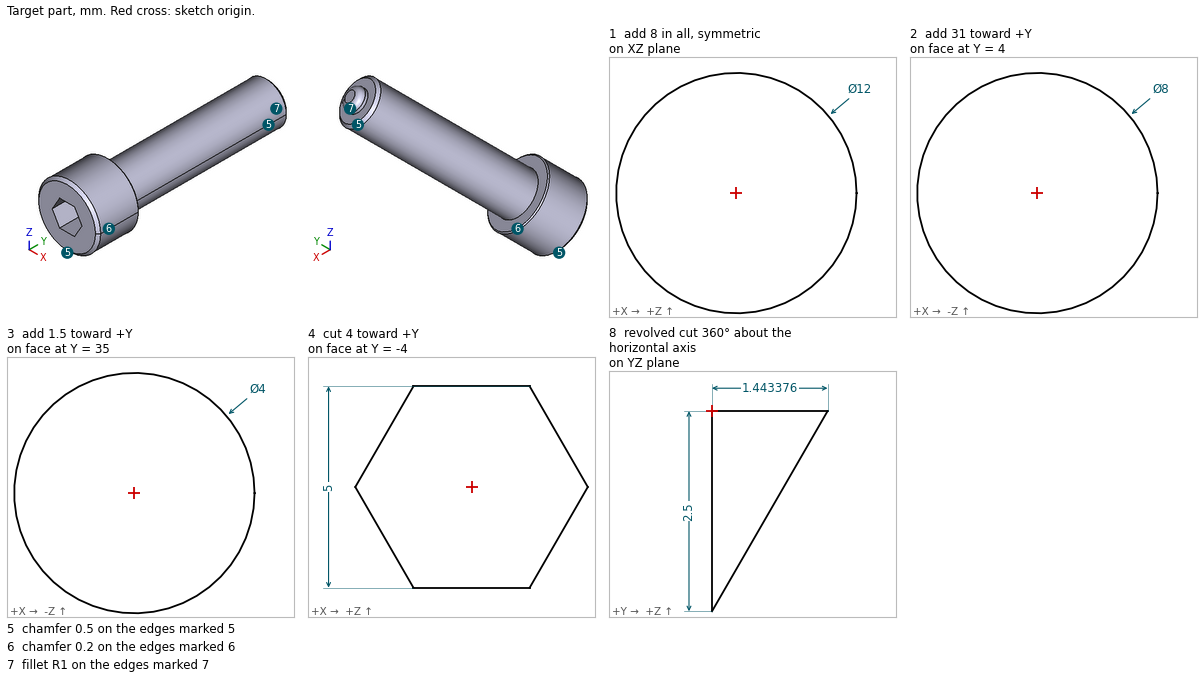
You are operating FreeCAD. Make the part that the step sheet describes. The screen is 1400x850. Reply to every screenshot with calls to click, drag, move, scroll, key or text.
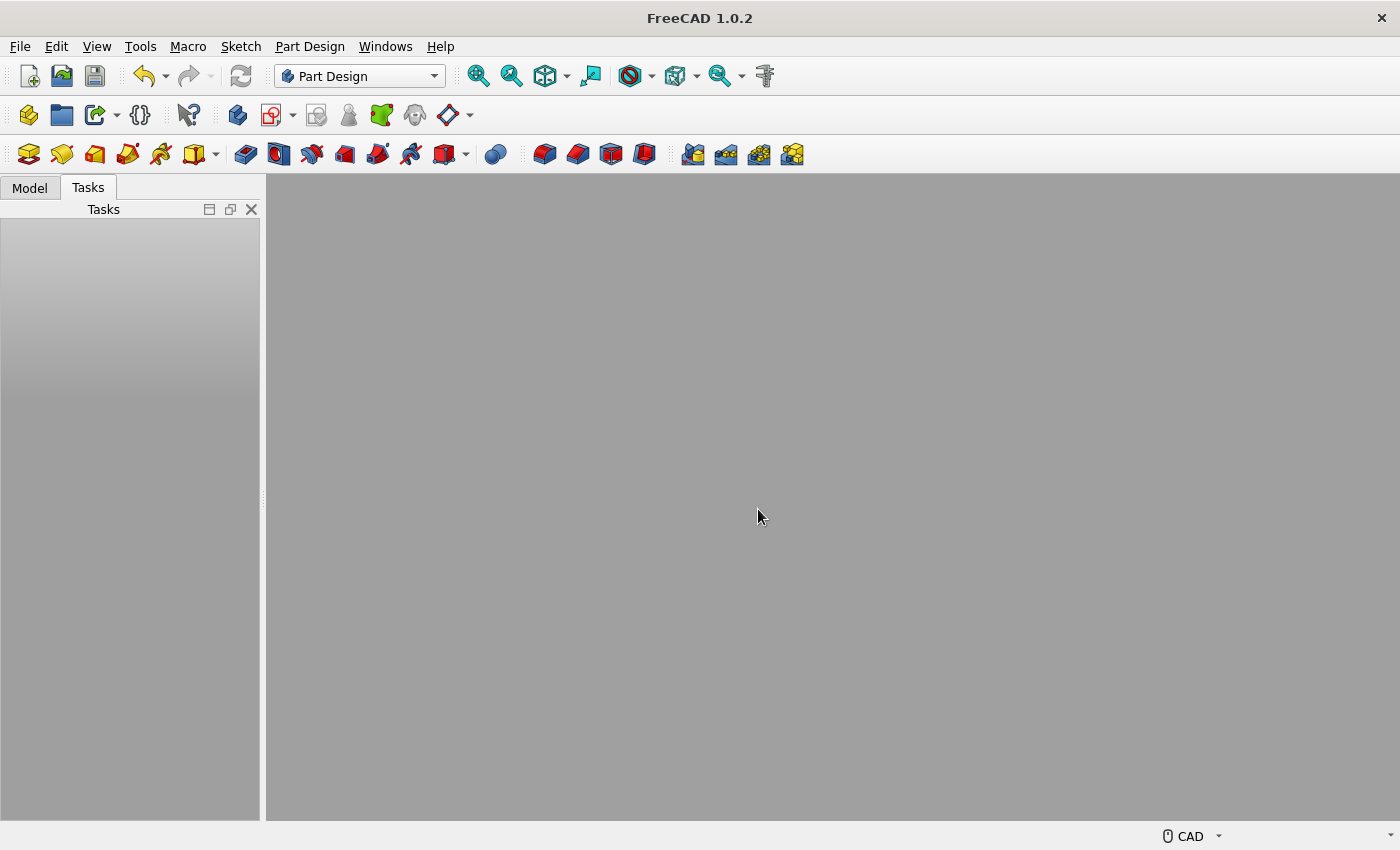
click(29, 76)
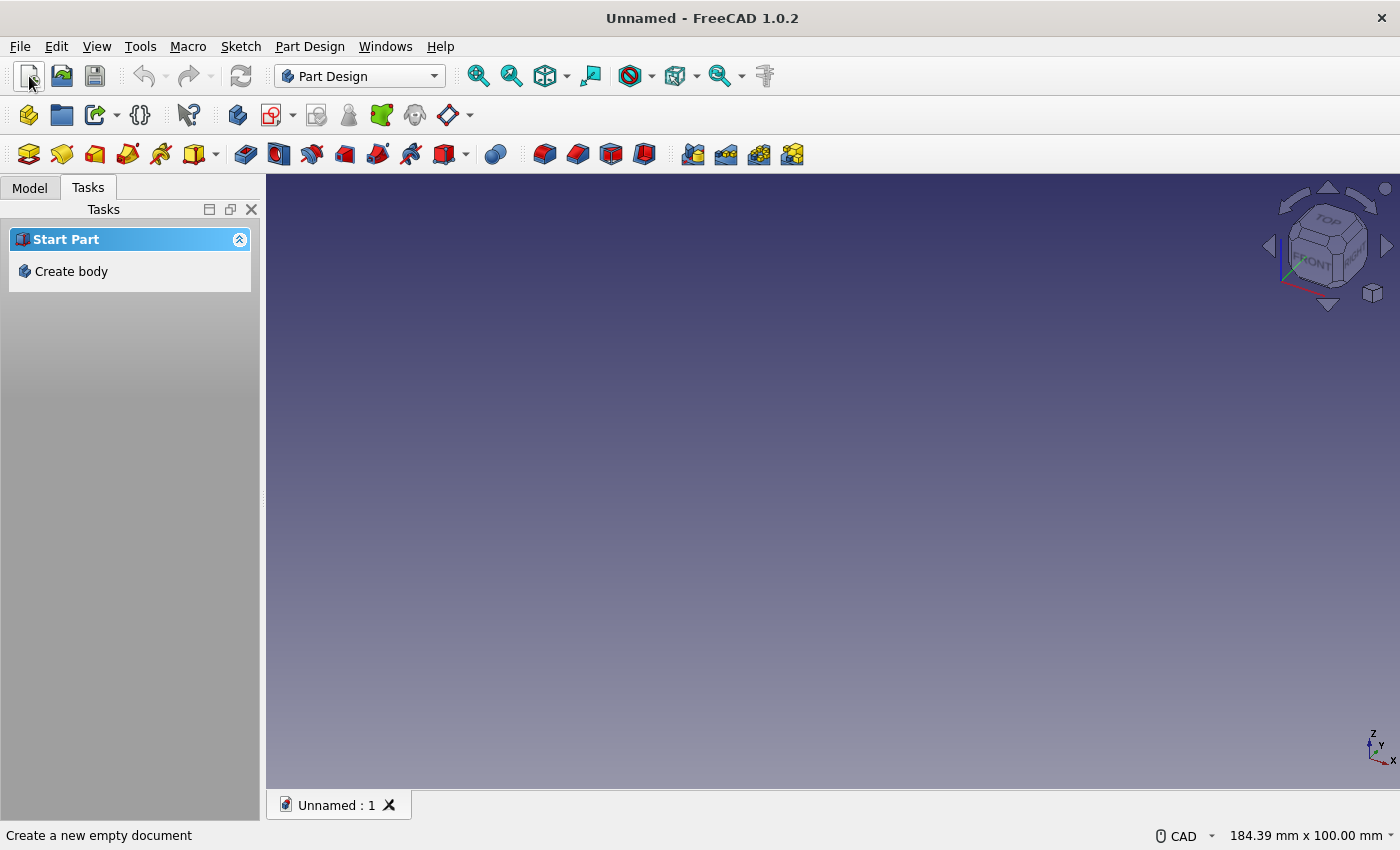
click(270, 116)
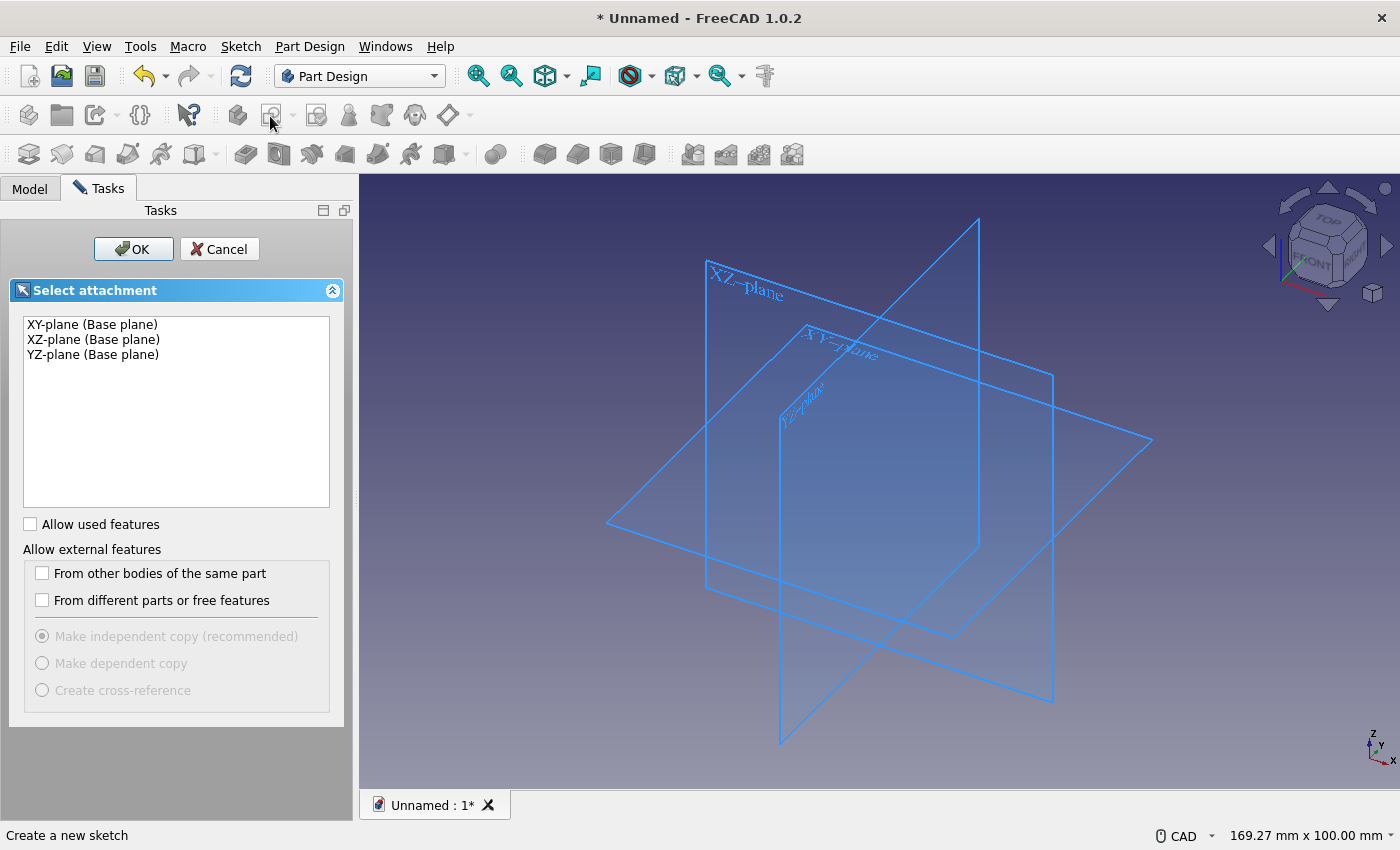
click(84, 340)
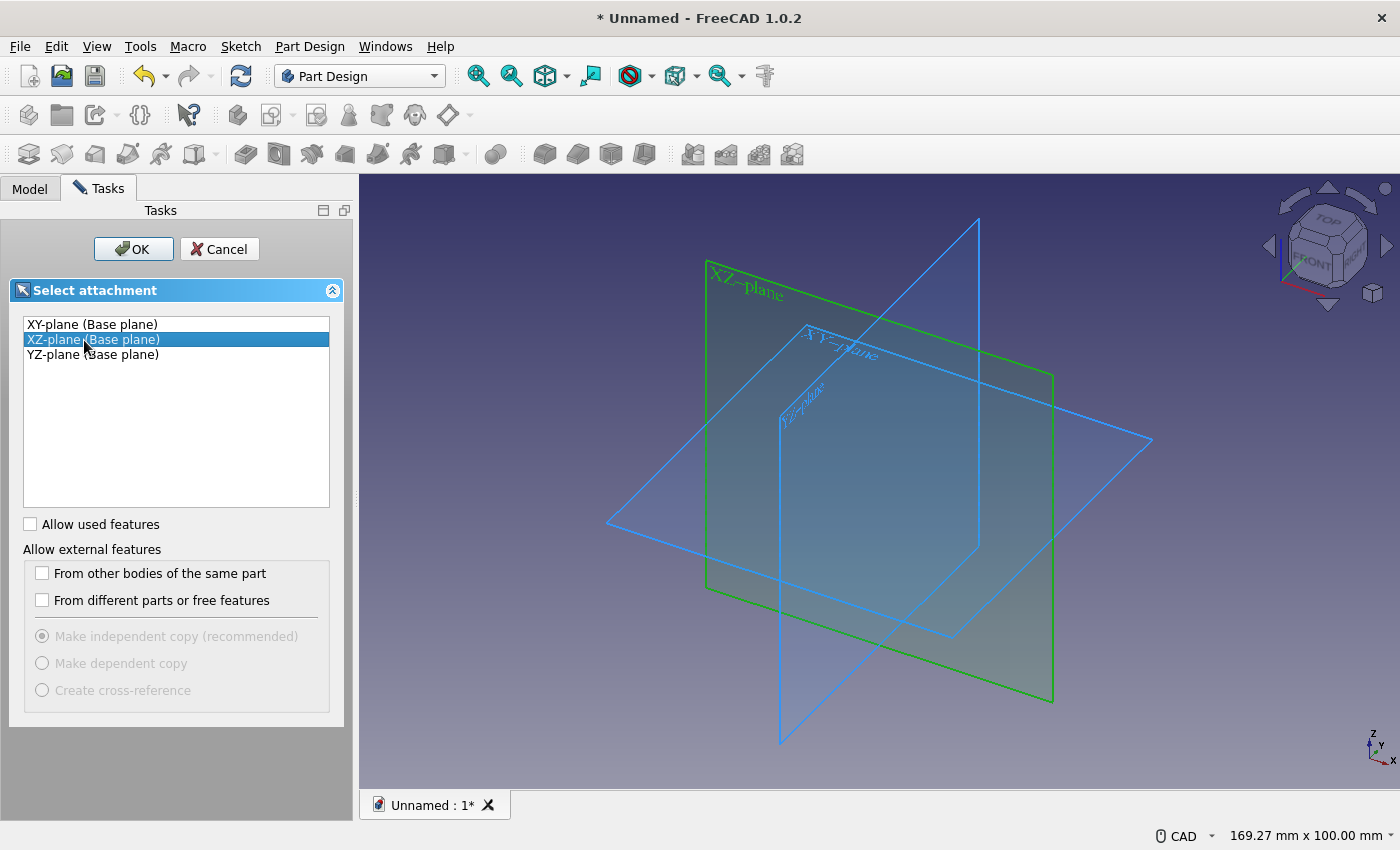
click(134, 249)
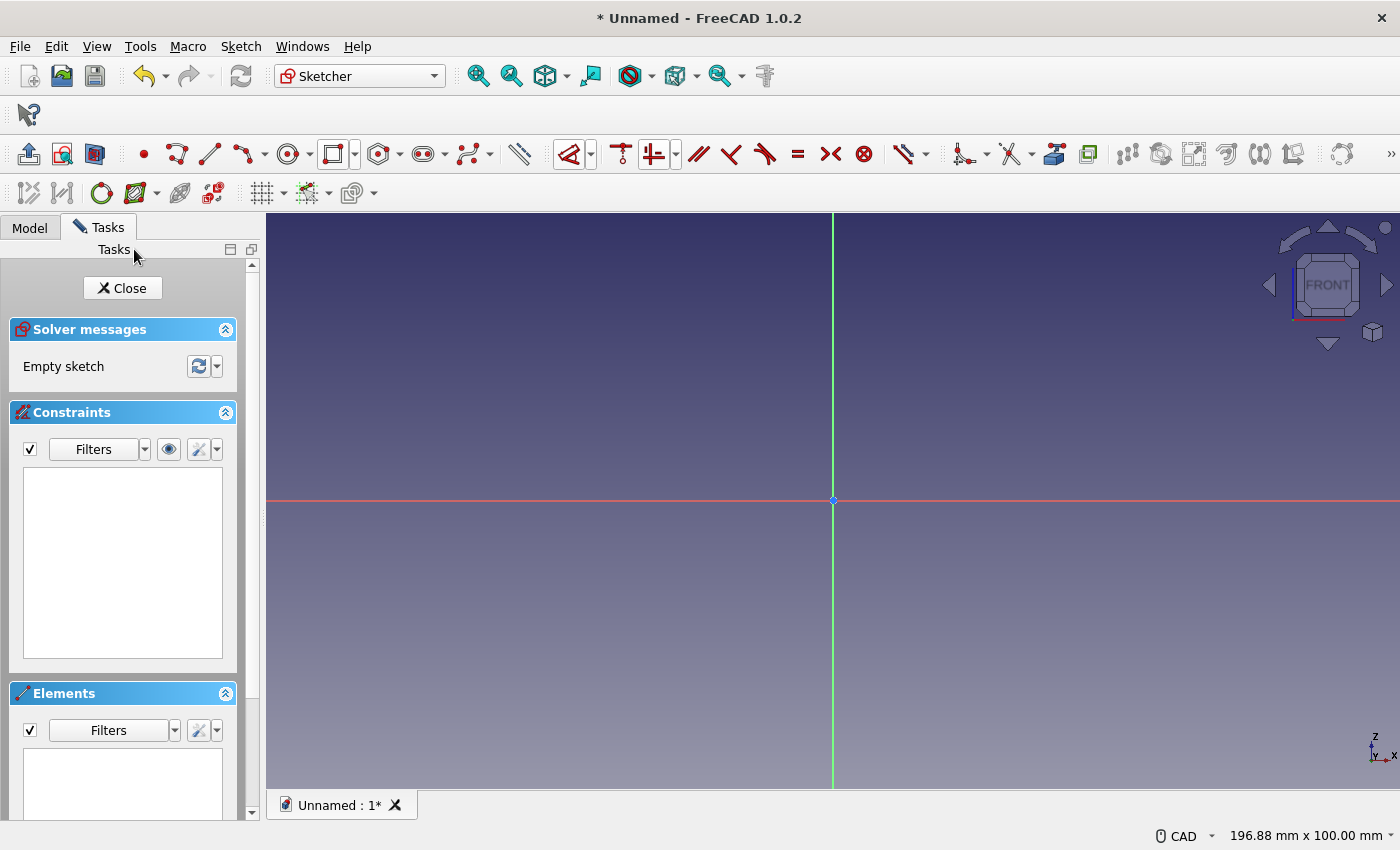
scroll(850, 501, up, 8)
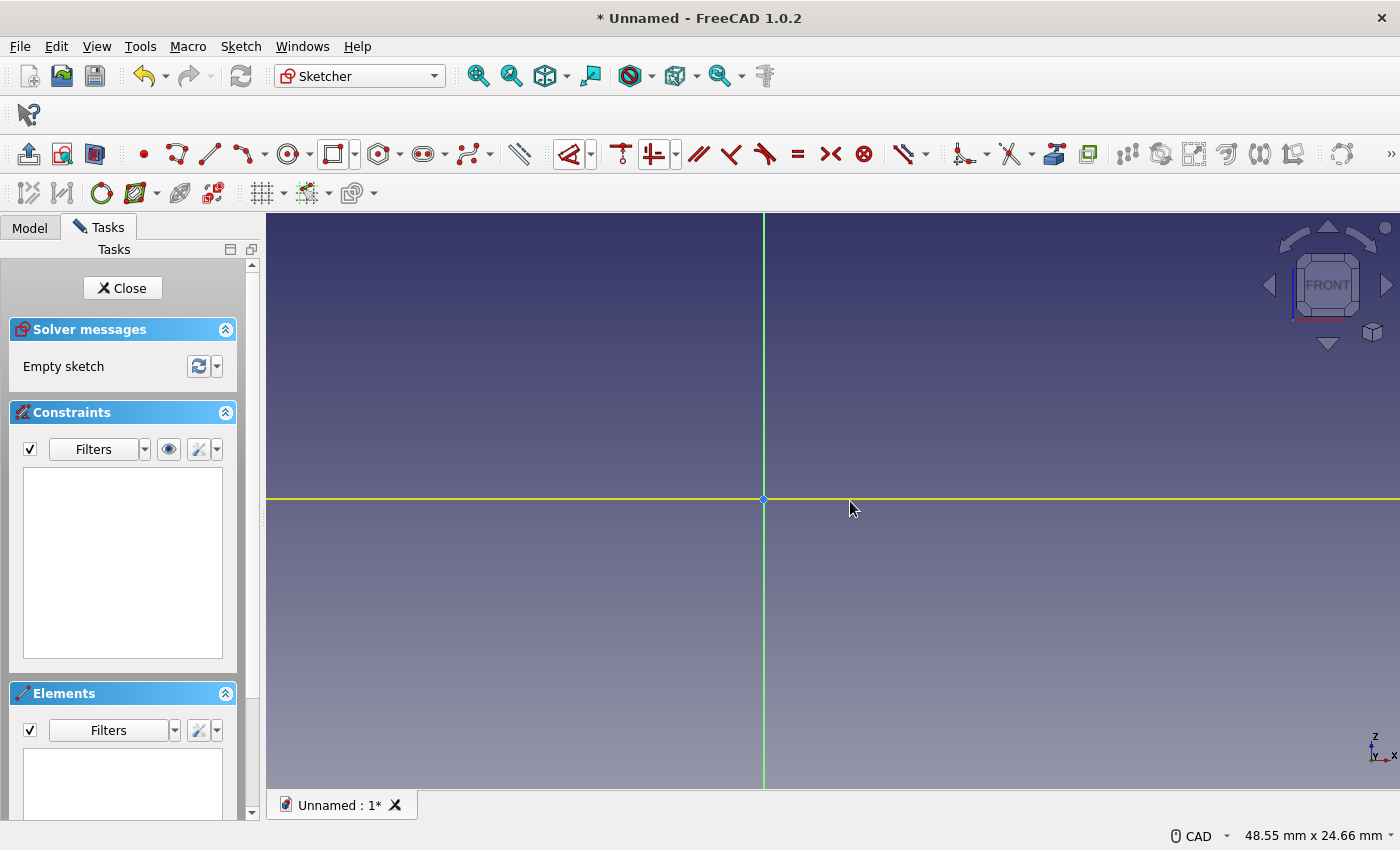
click(288, 154)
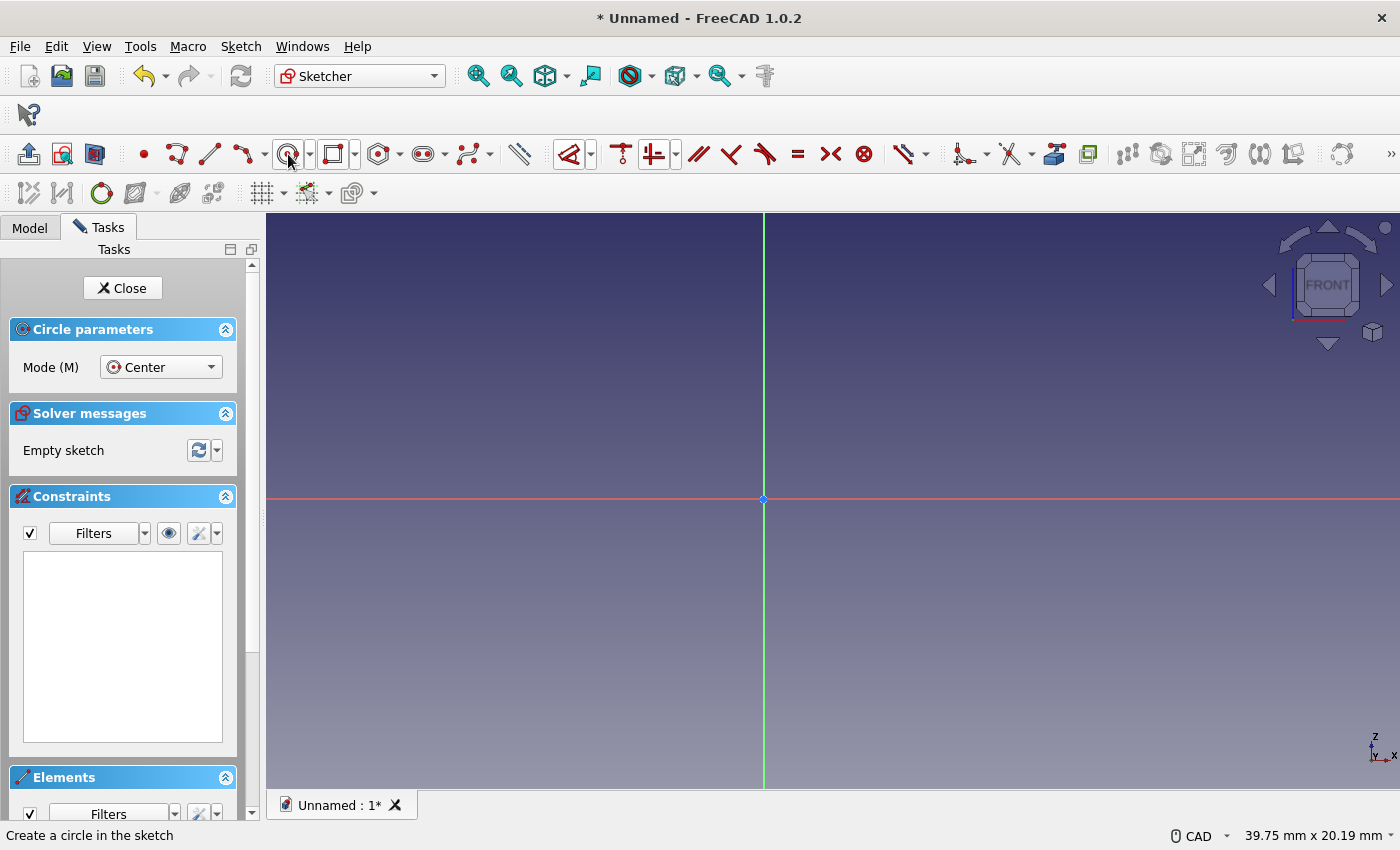
click(764, 499)
move(885, 378)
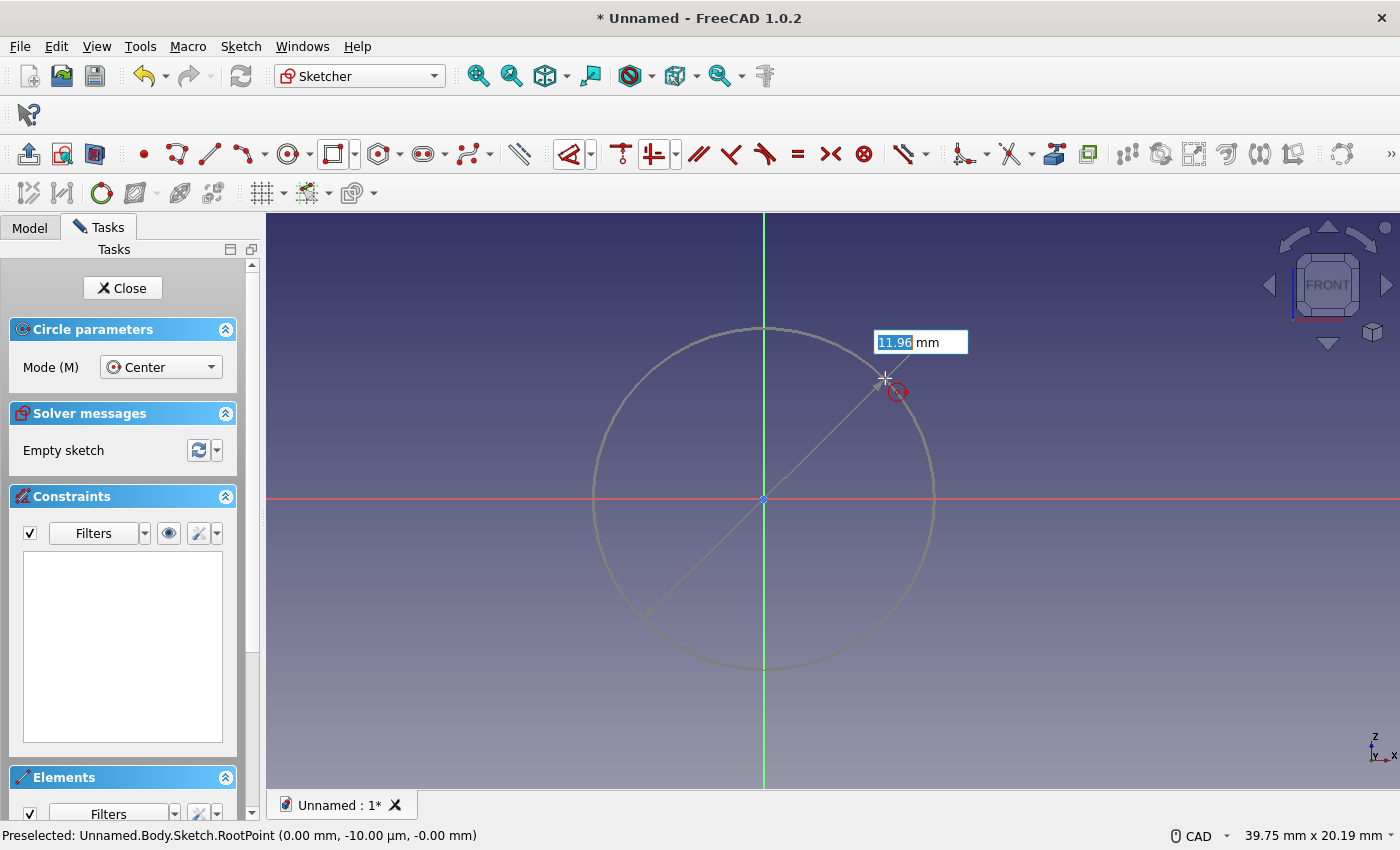
text(12)
key(Return)
key(Escape)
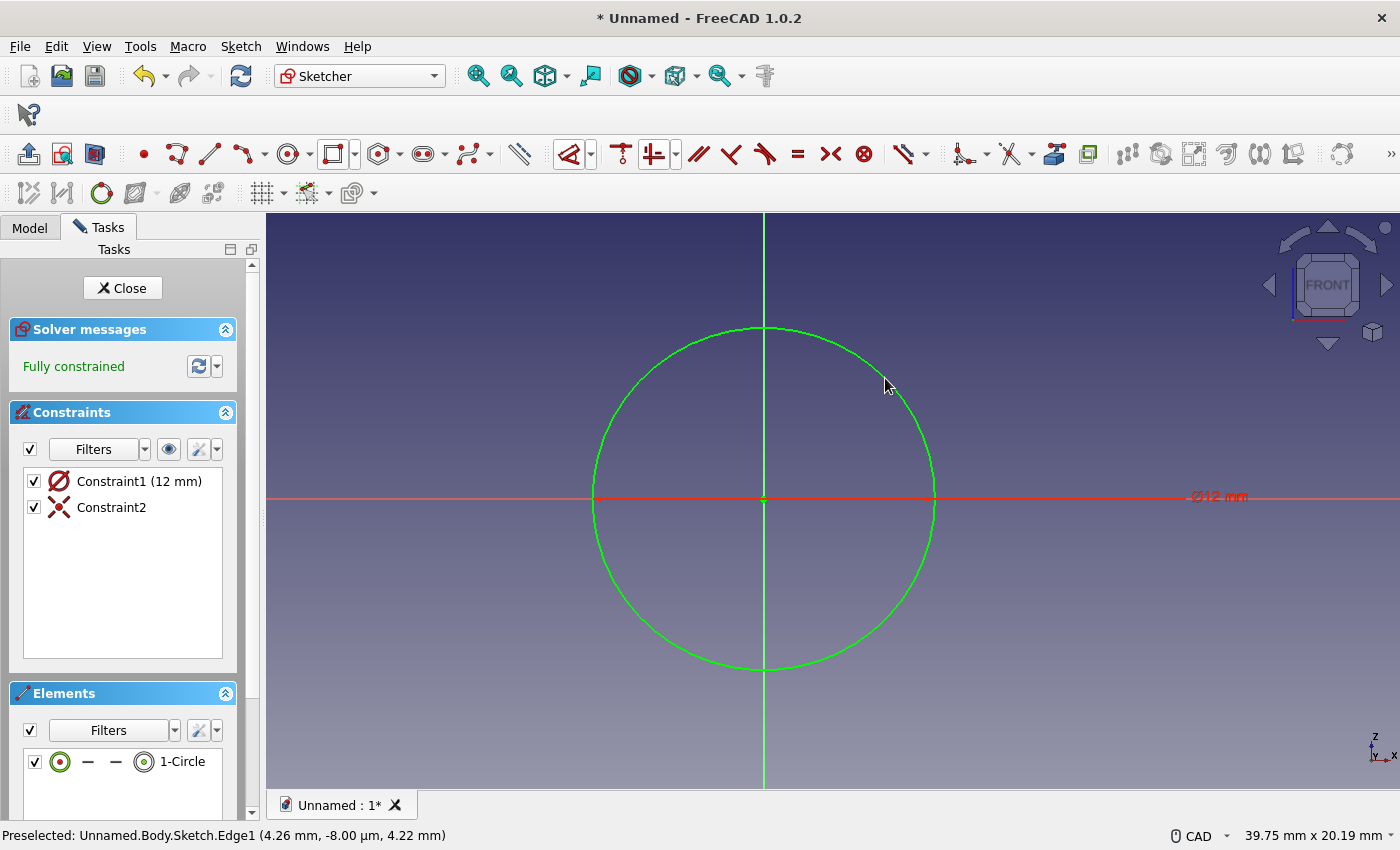
click(123, 288)